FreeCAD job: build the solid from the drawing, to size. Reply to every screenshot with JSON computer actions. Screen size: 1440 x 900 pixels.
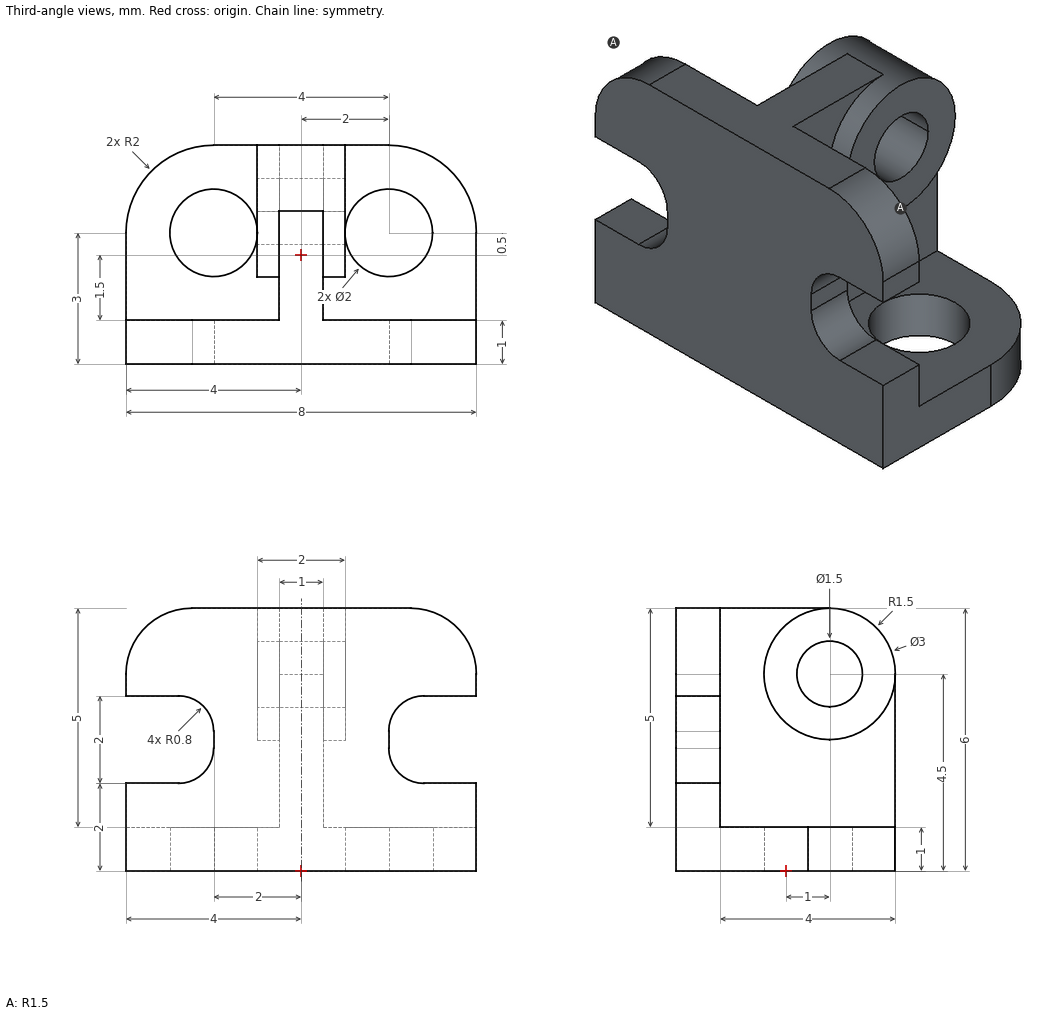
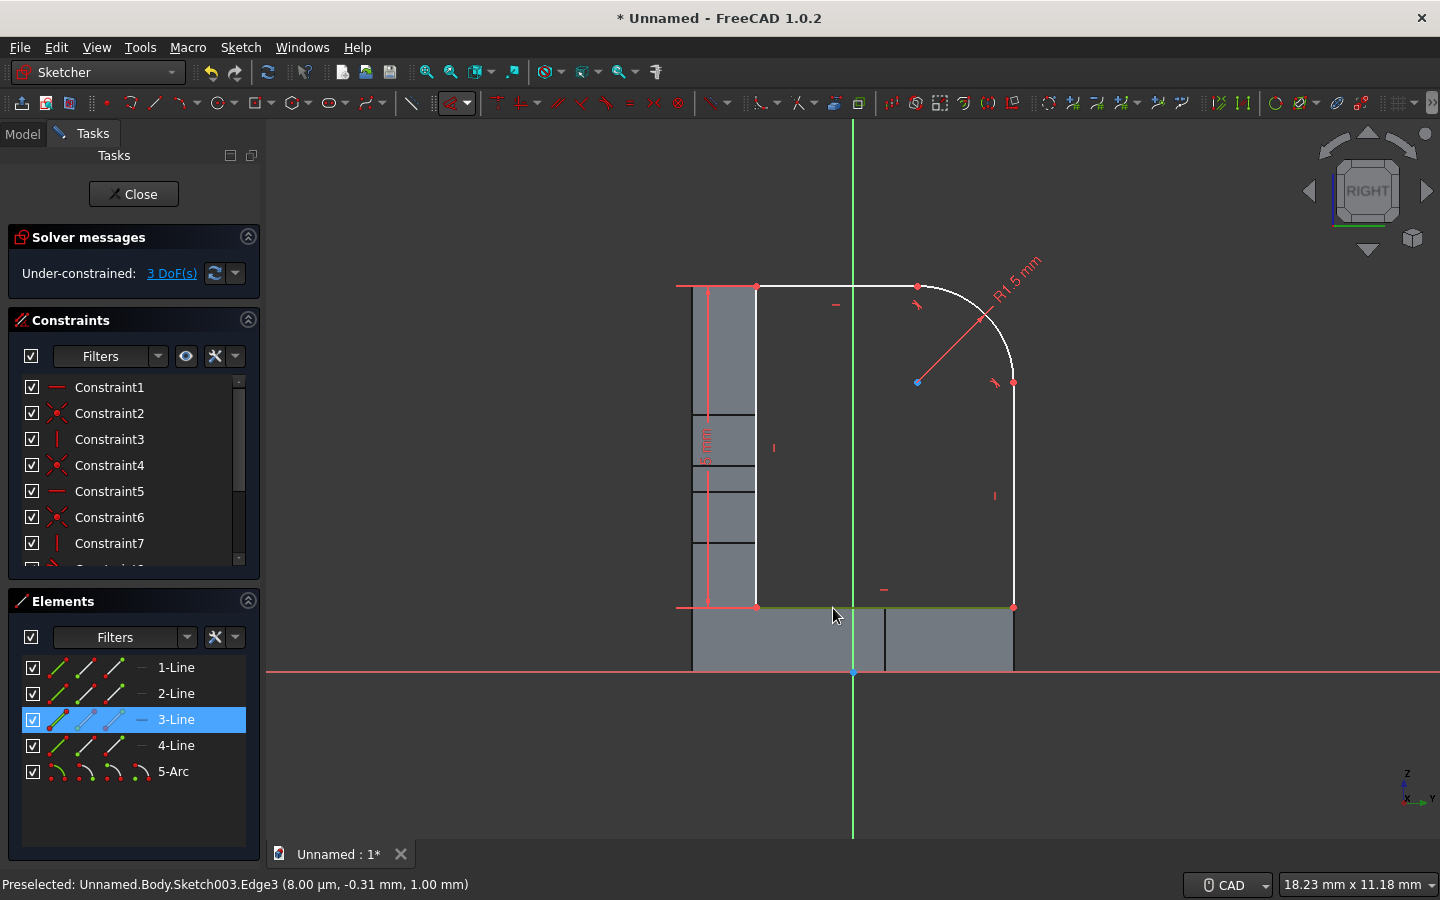
{"action": "key", "text": "l"}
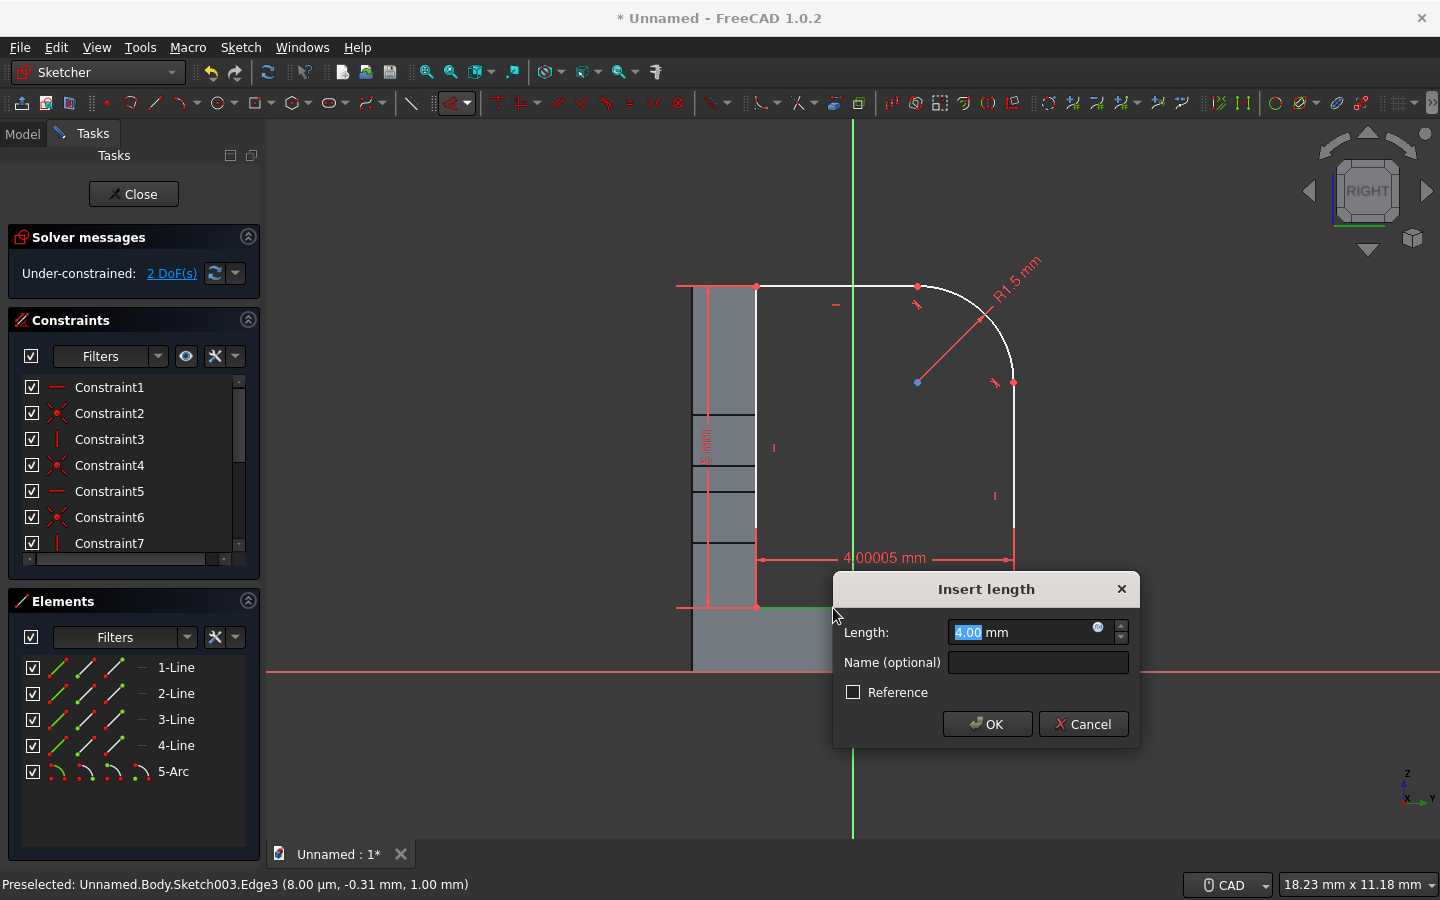
{"action": "type", "text": "4"}
{"action": "key", "text": "Return"}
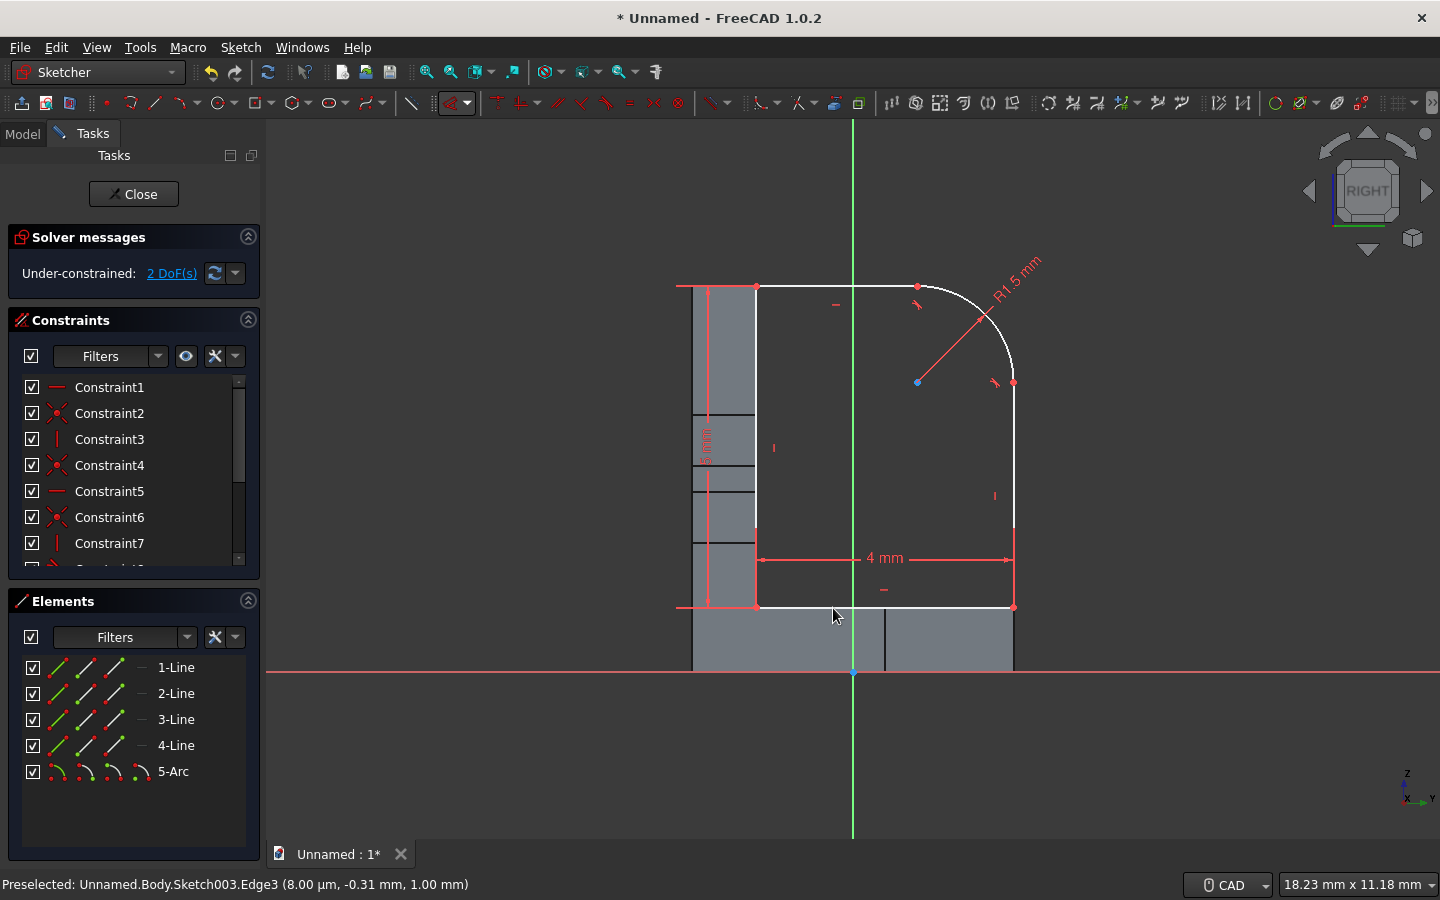
{"action": "left_click", "coordinate": [917, 286]}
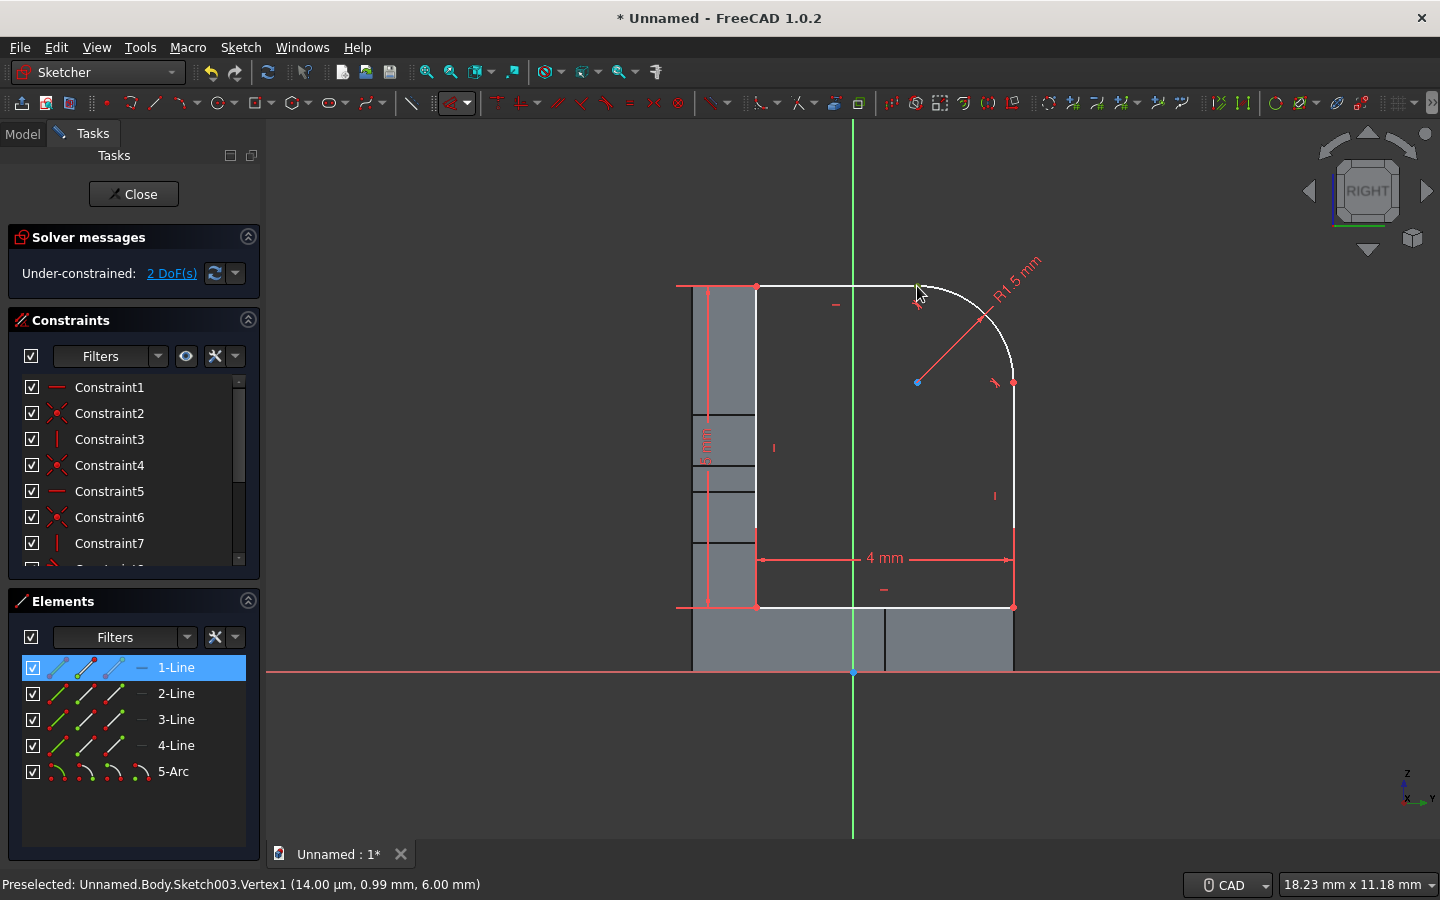
{"action": "key", "text": "l"}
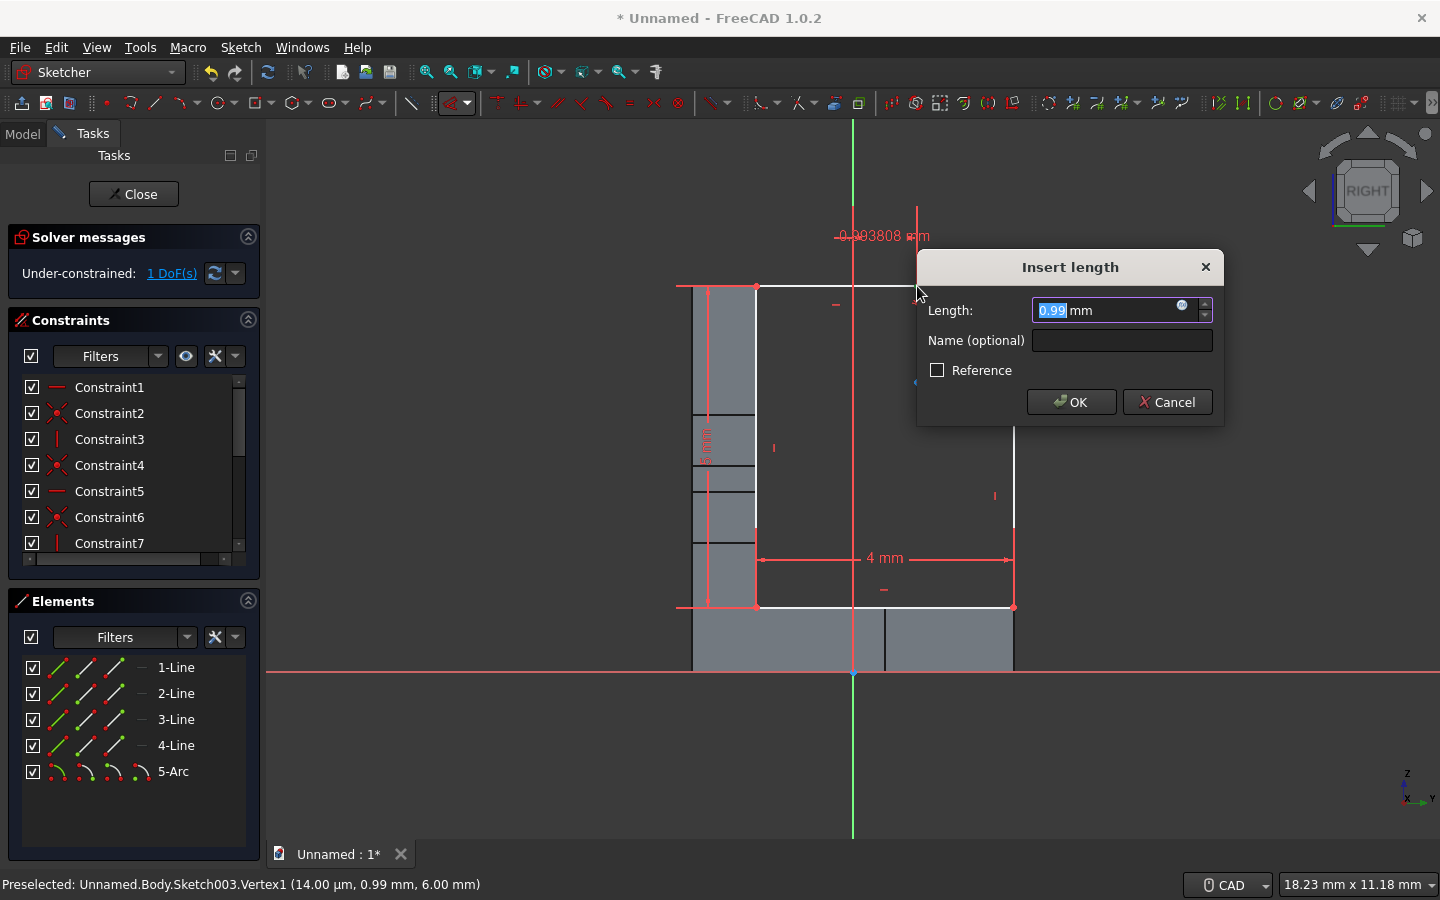
{"action": "type", "text": "1"}
{"action": "key", "text": "Return"}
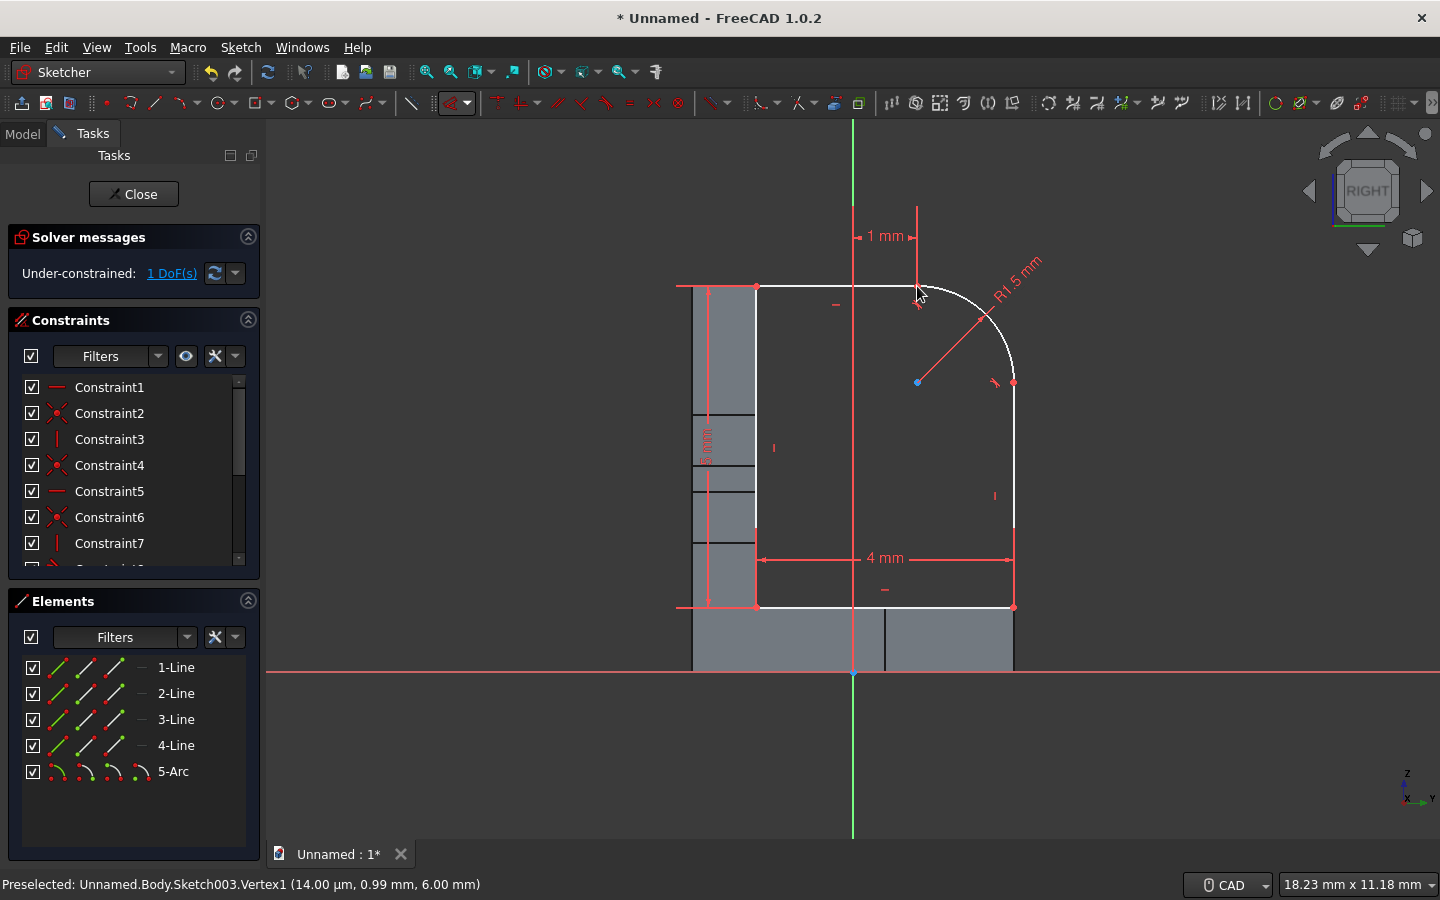
{"action": "left_click", "coordinate": [917, 286]}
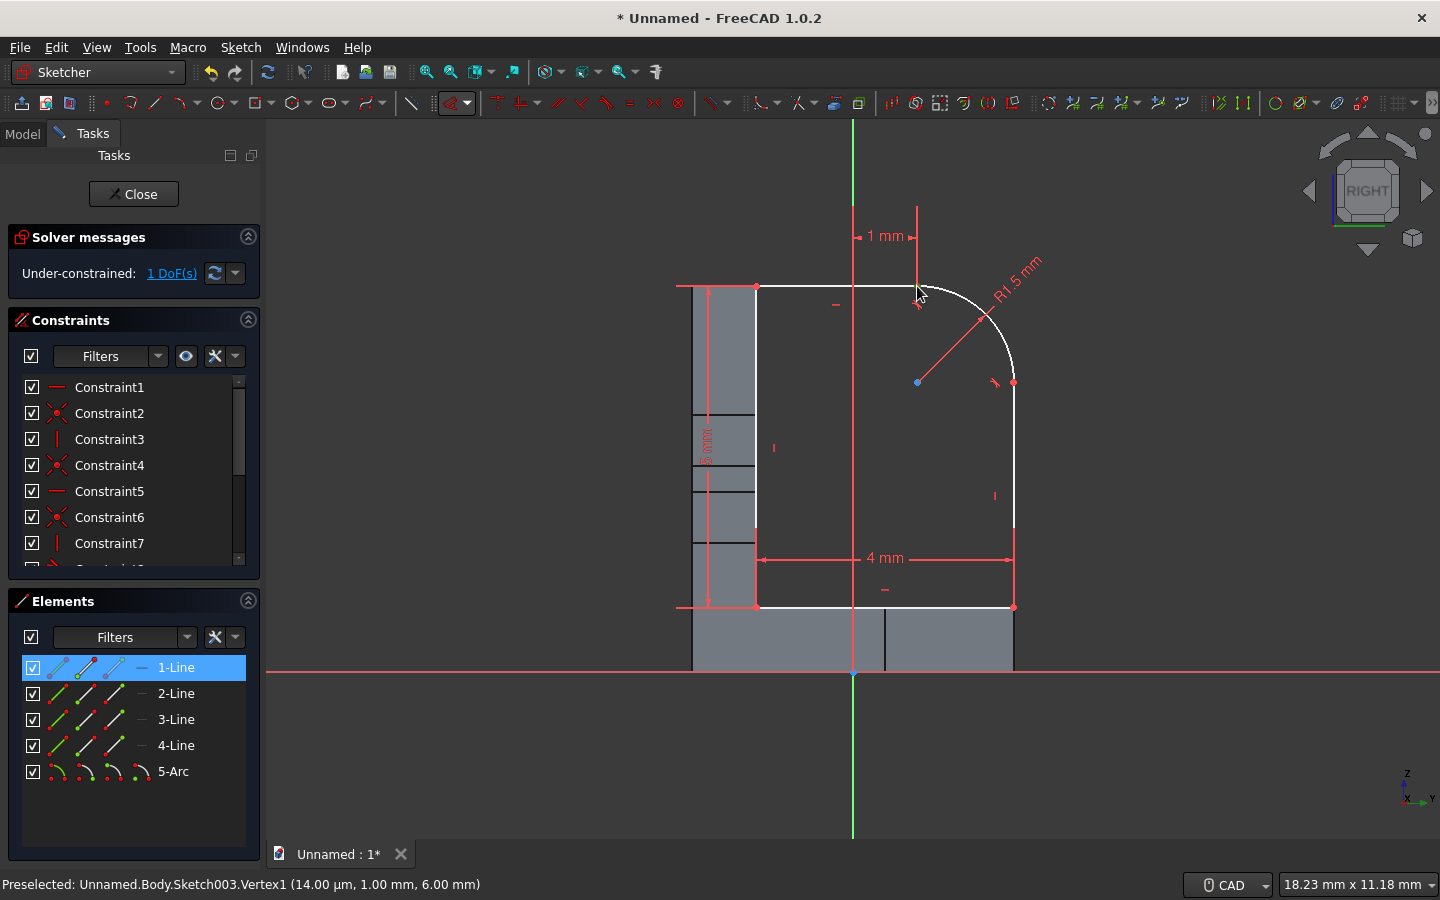
{"action": "key", "text": "i"}